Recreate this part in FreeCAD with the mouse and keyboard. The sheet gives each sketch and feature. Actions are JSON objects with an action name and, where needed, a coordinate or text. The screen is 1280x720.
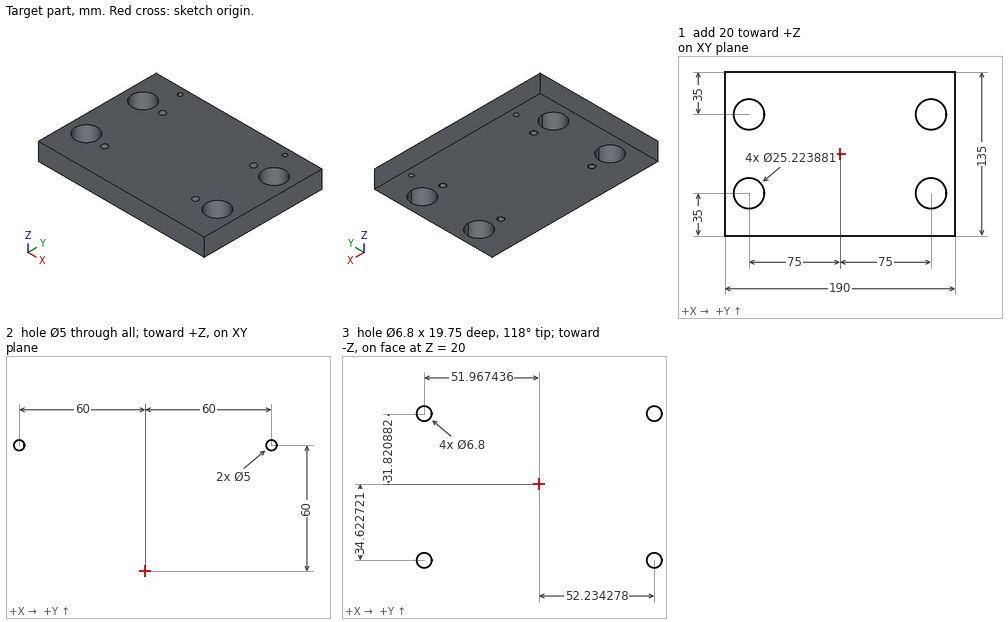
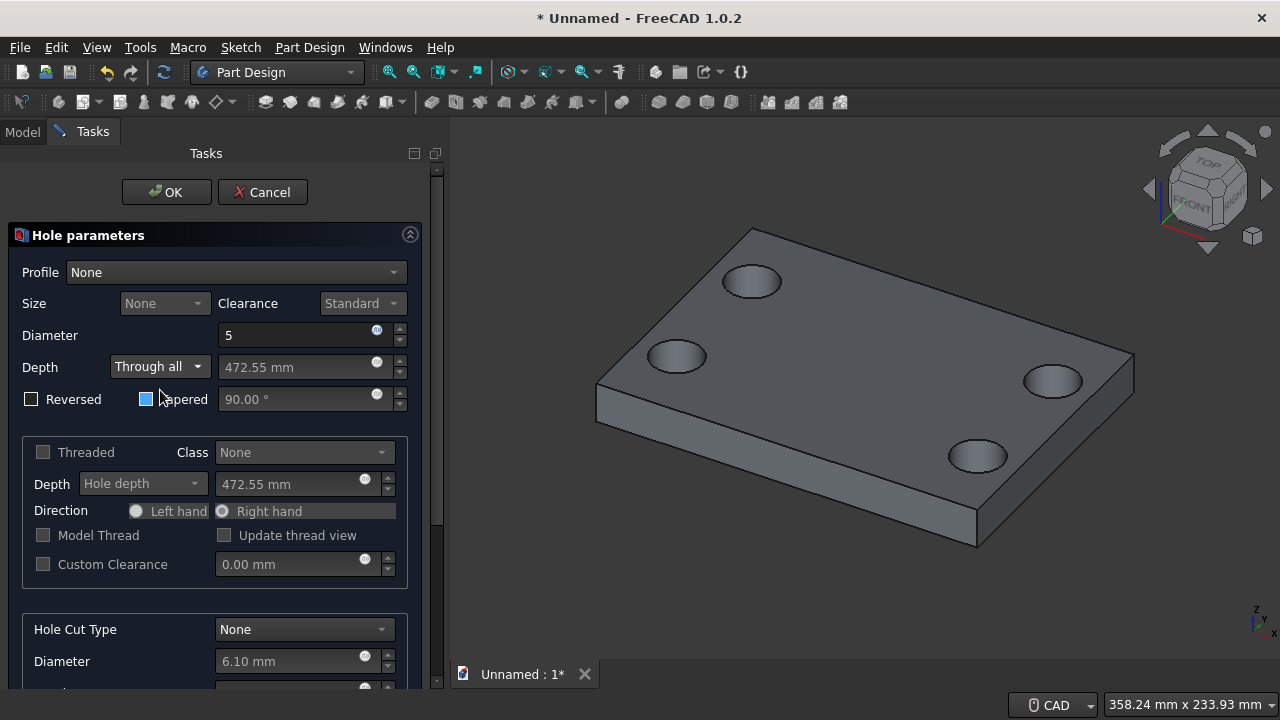
{"action": "left_click", "coordinate": [30, 399]}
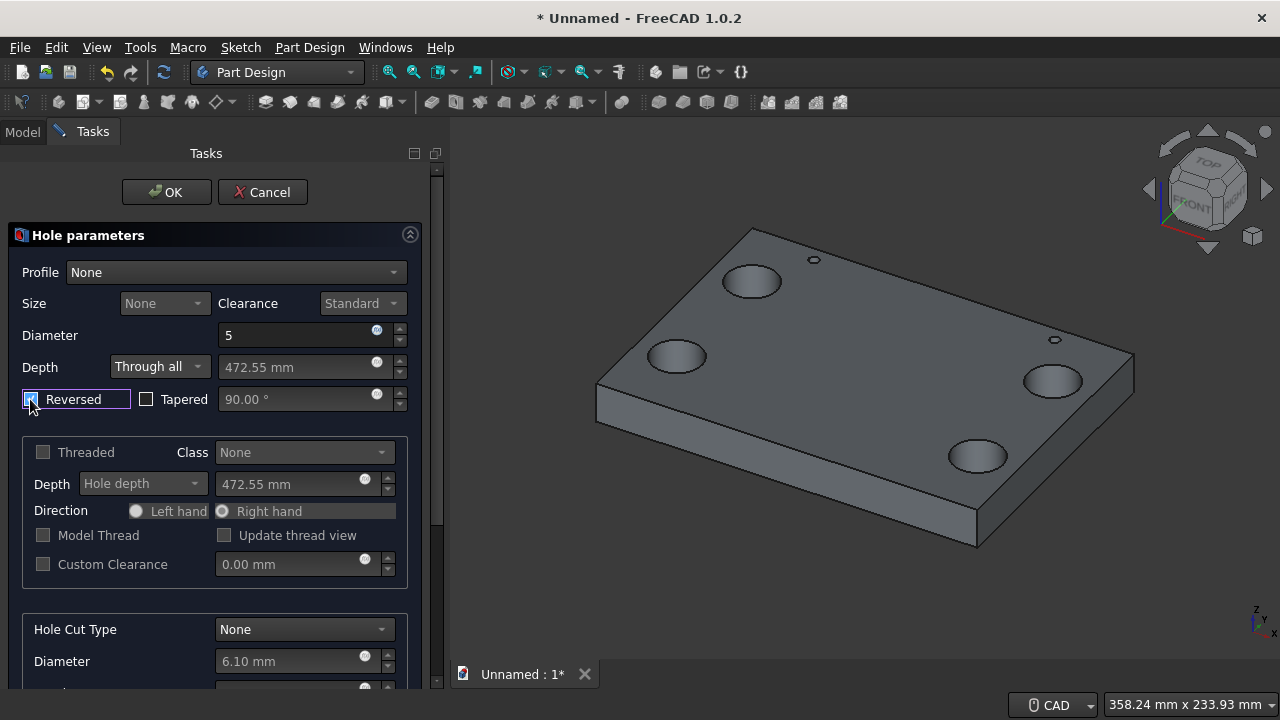
{"action": "left_click", "coordinate": [167, 192]}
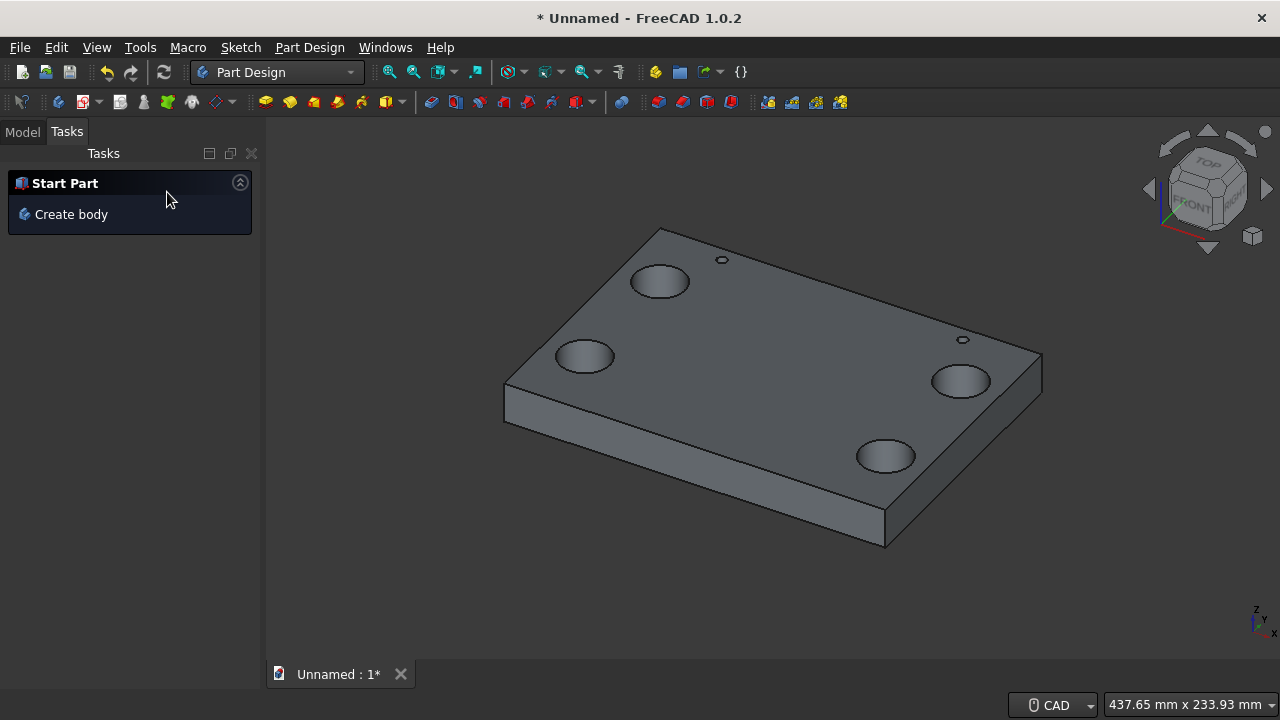
{"action": "left_click", "coordinate": [773, 368]}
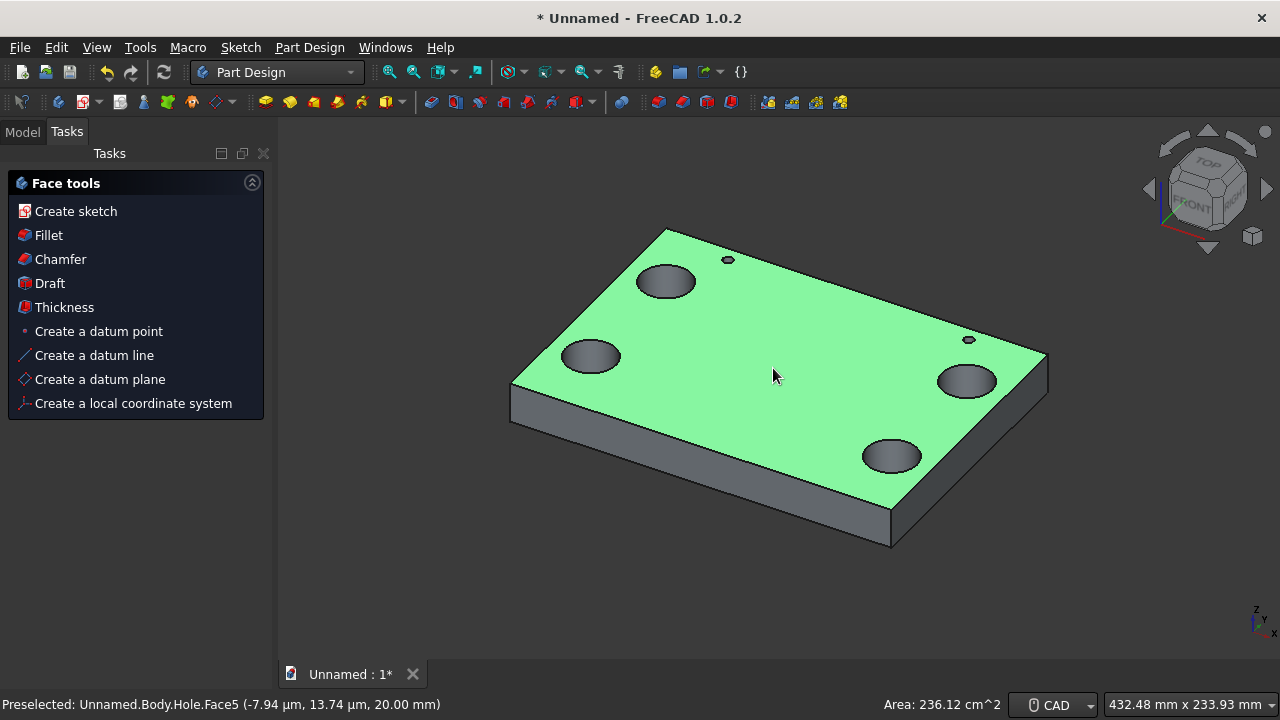
{"action": "left_click", "coordinate": [84, 102]}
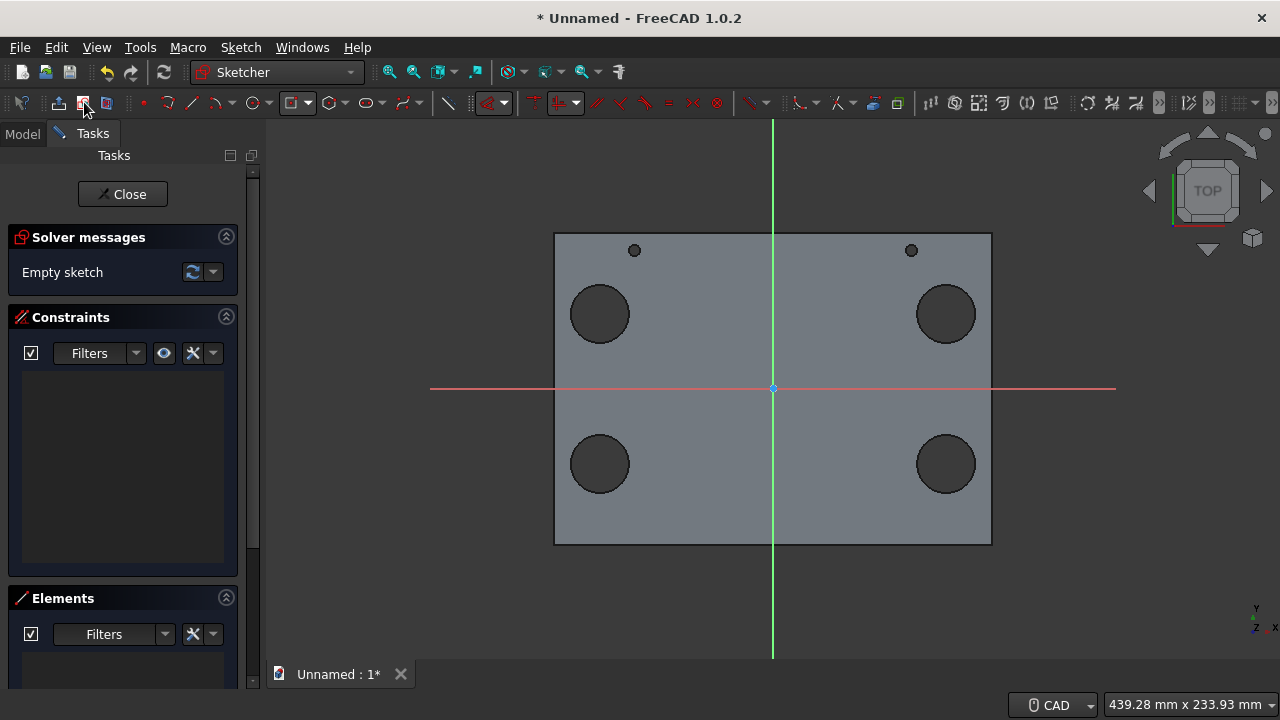
{"action": "scroll", "coordinate": [829, 395], "scroll_direction": "up", "scroll_amount": 4}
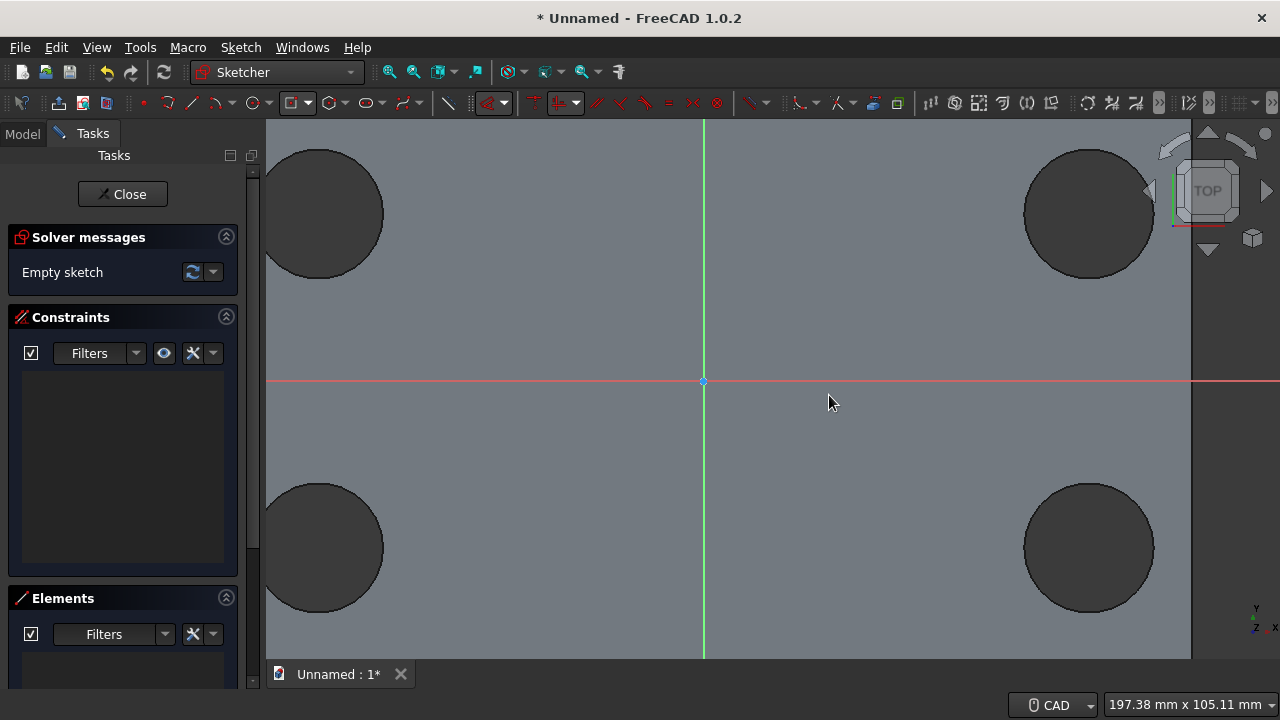
{"action": "left_click", "coordinate": [254, 104]}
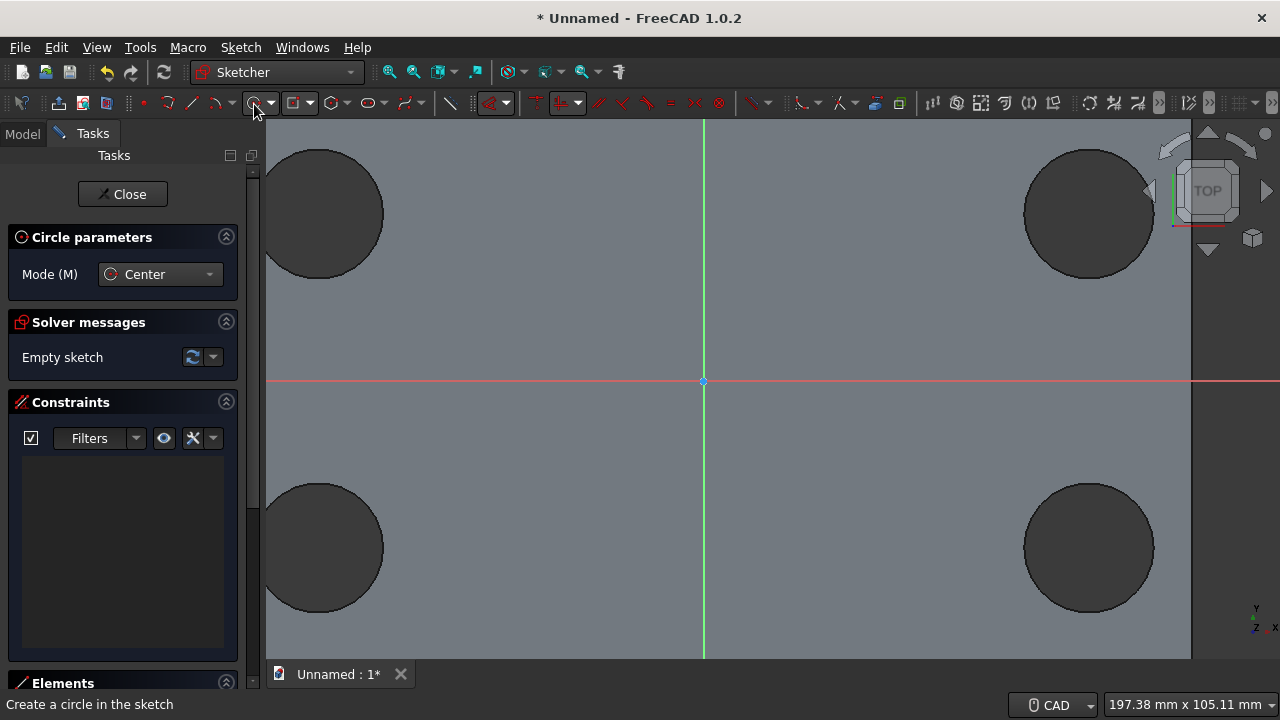
{"action": "scroll", "coordinate": [437, 218], "scroll_direction": "up", "scroll_amount": 2}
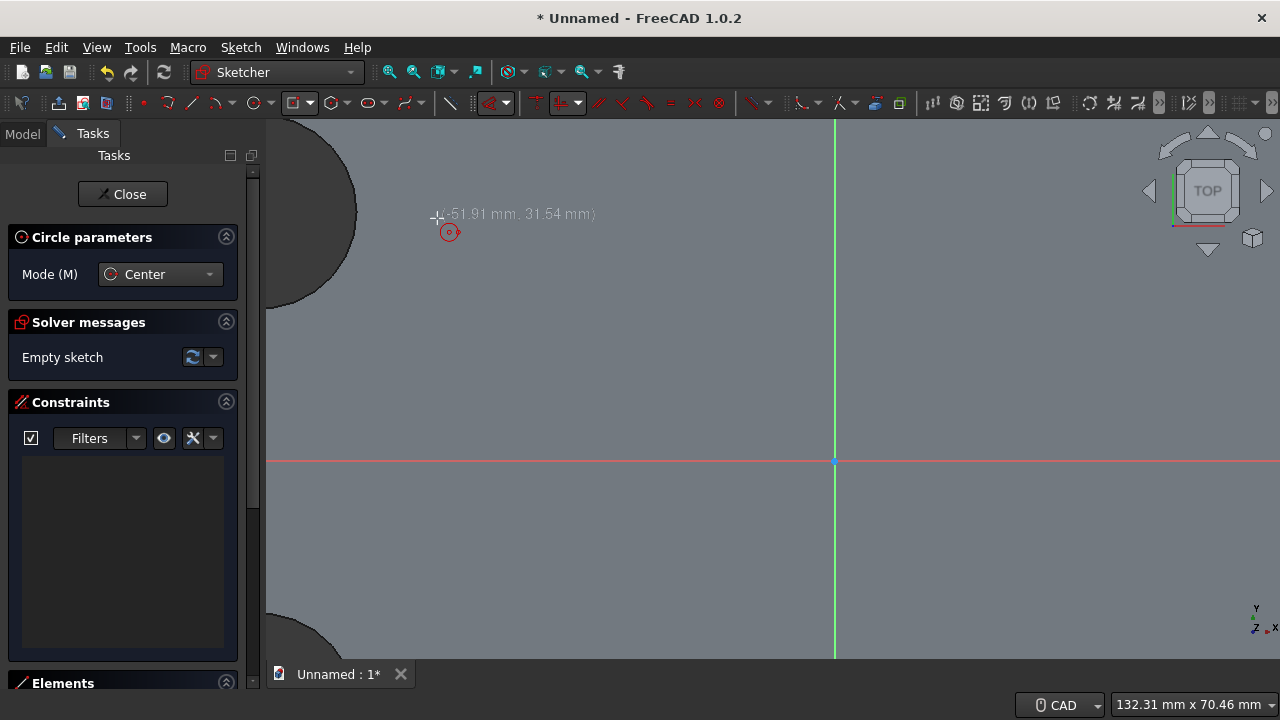
{"action": "left_click", "coordinate": [436, 217]}
{"action": "mouse_move", "coordinate": [455, 199]}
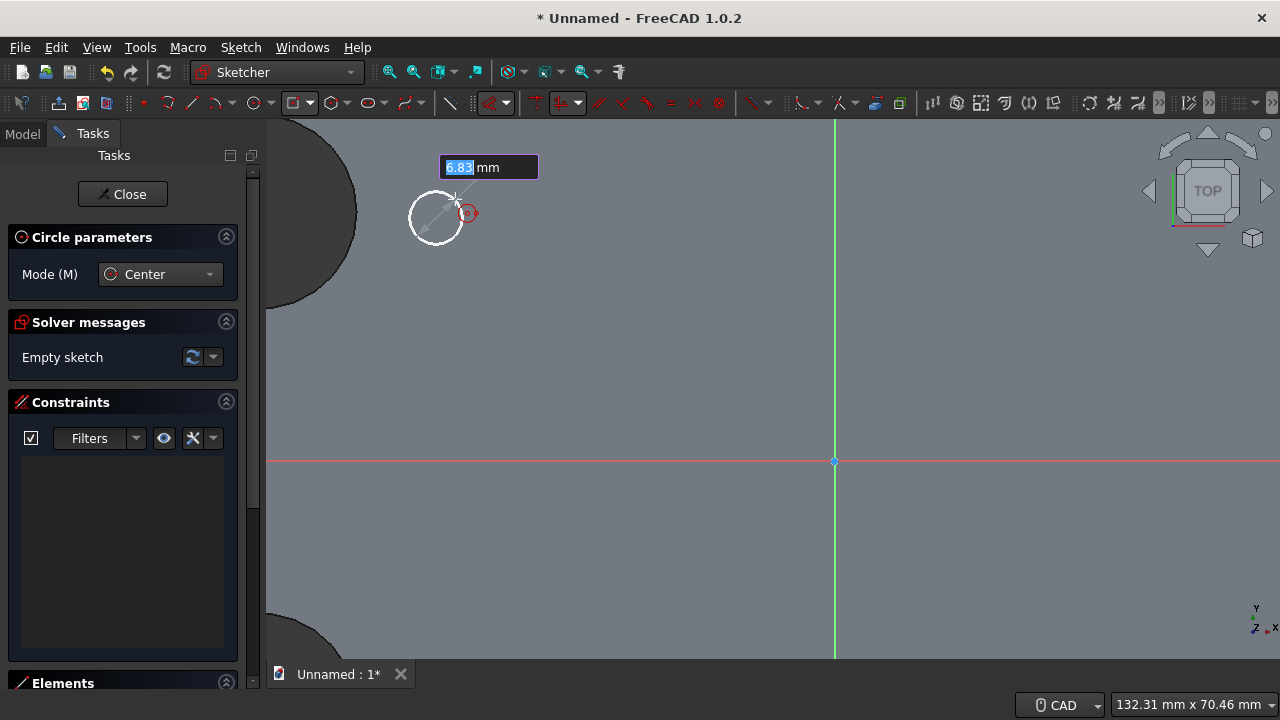
{"action": "type", "text": "6.8"}
{"action": "key", "text": "Return"}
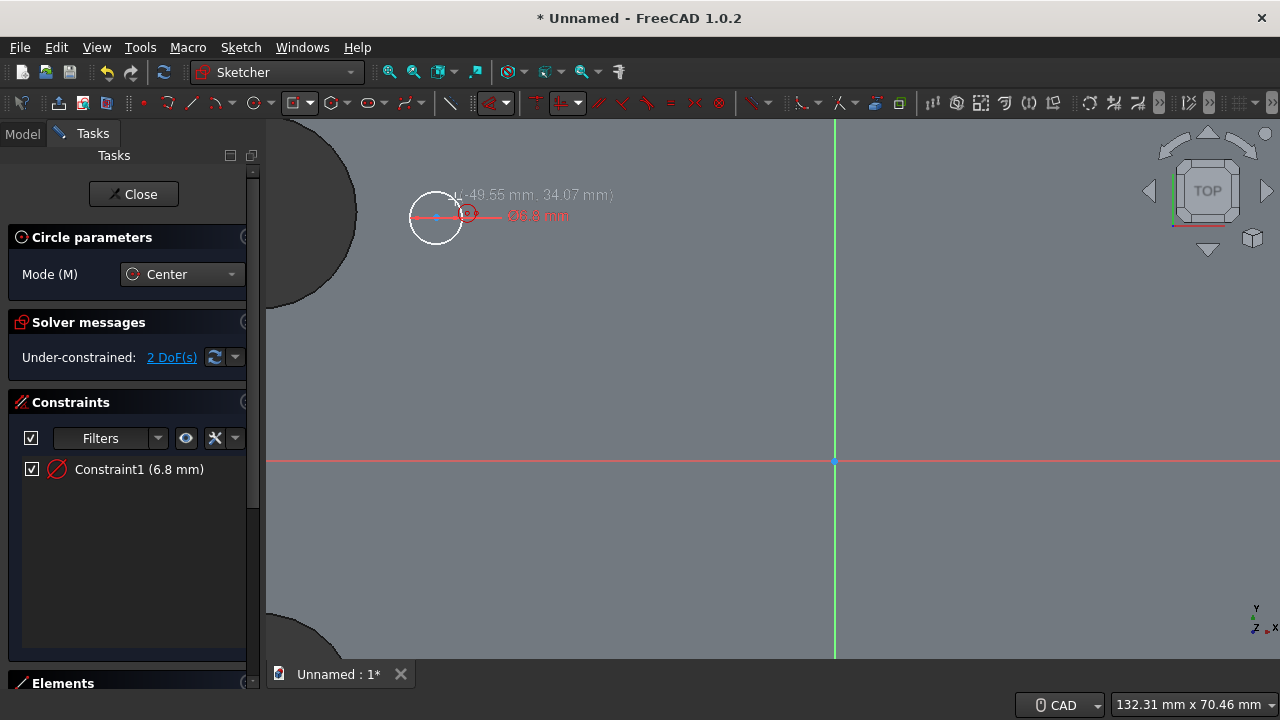
{"action": "scroll", "coordinate": [438, 221], "scroll_direction": "down", "scroll_amount": 2}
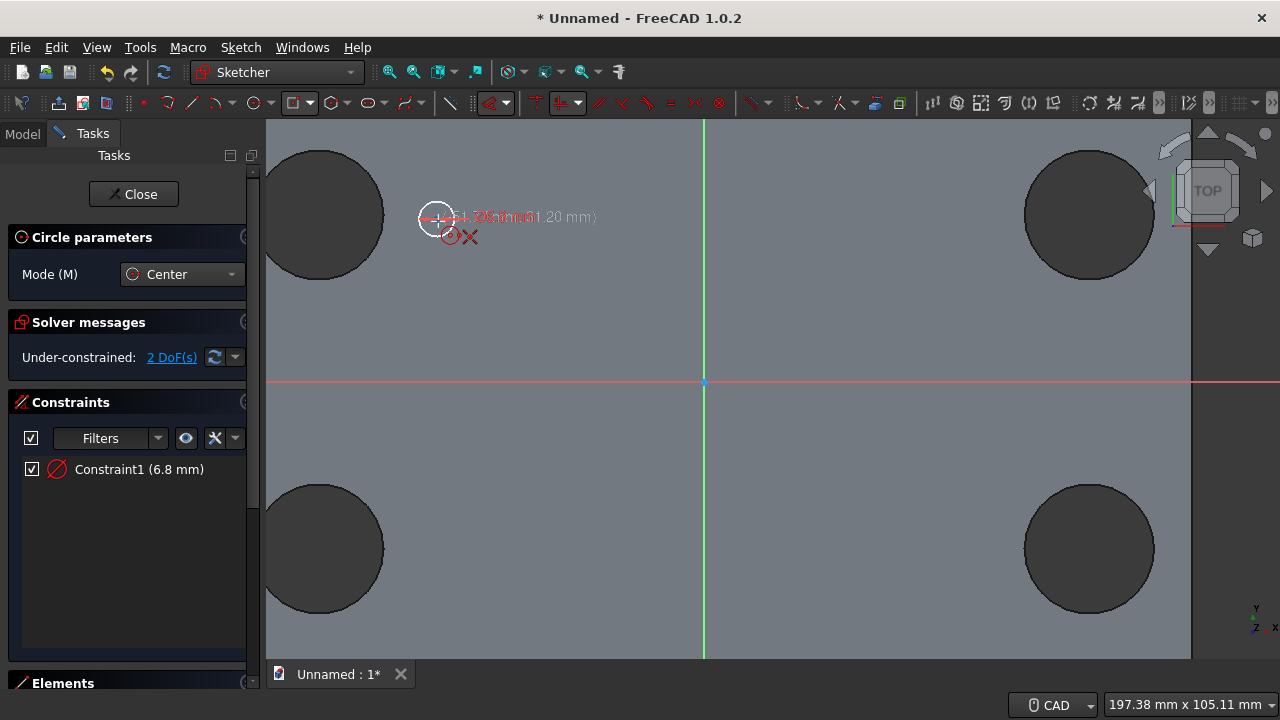
{"action": "scroll", "coordinate": [437, 560], "scroll_direction": "up", "scroll_amount": 2}